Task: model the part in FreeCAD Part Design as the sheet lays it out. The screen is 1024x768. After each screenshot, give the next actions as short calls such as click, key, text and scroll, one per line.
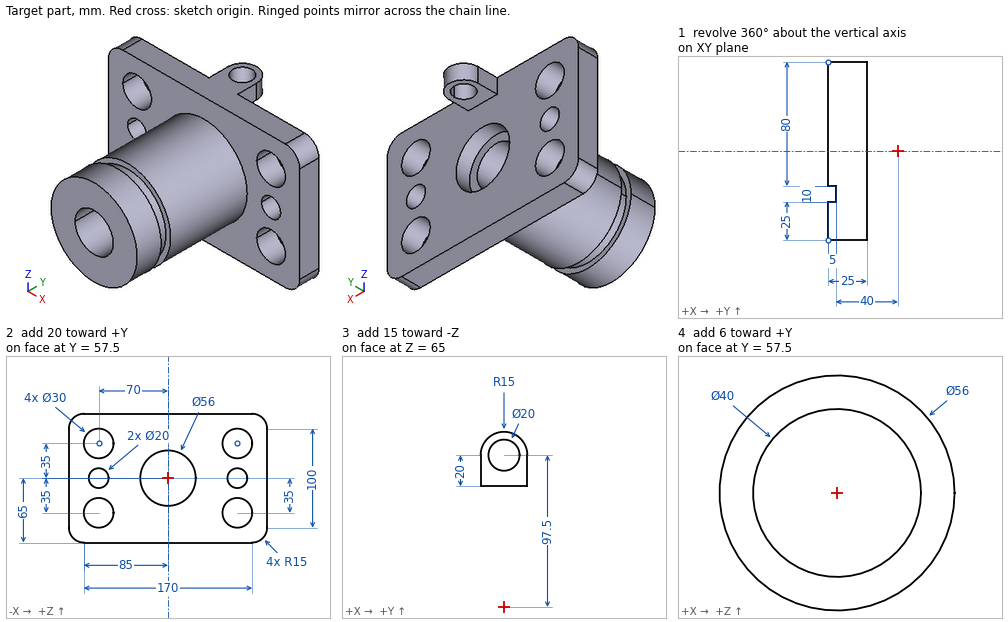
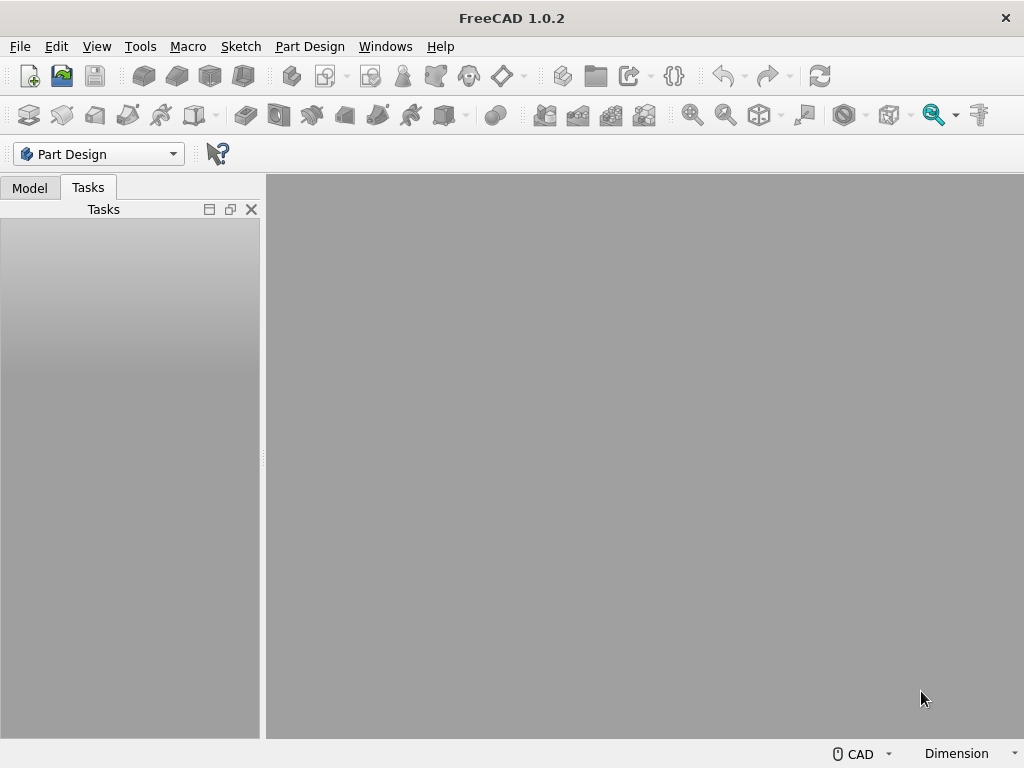
click(29, 76)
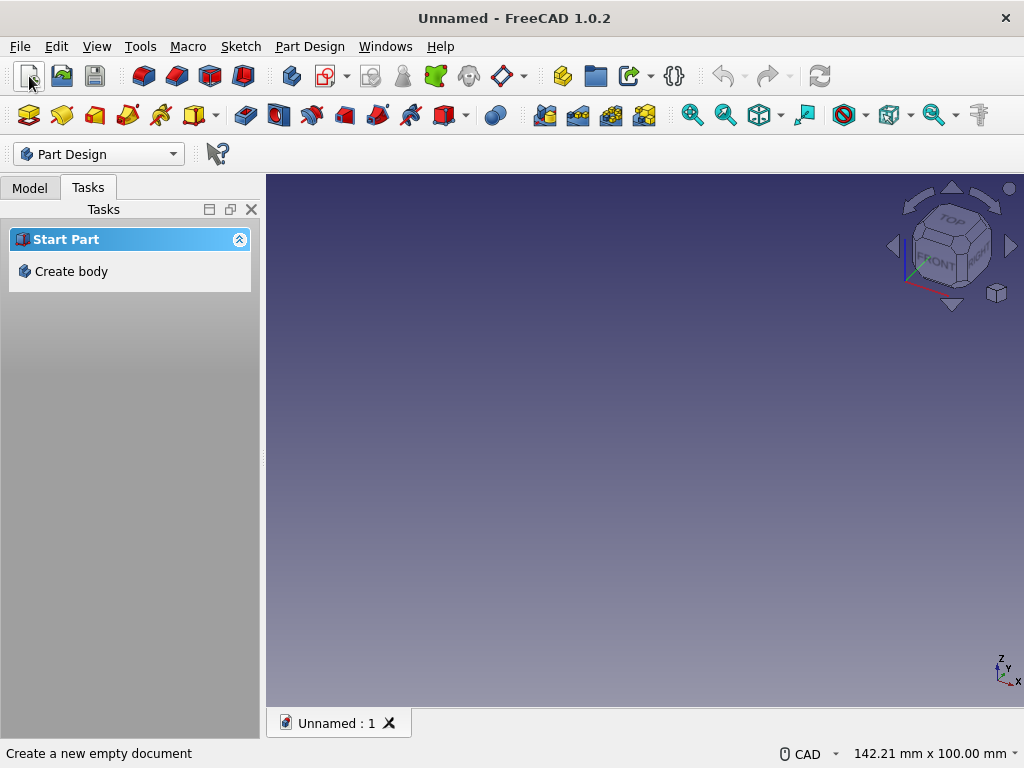
click(324, 76)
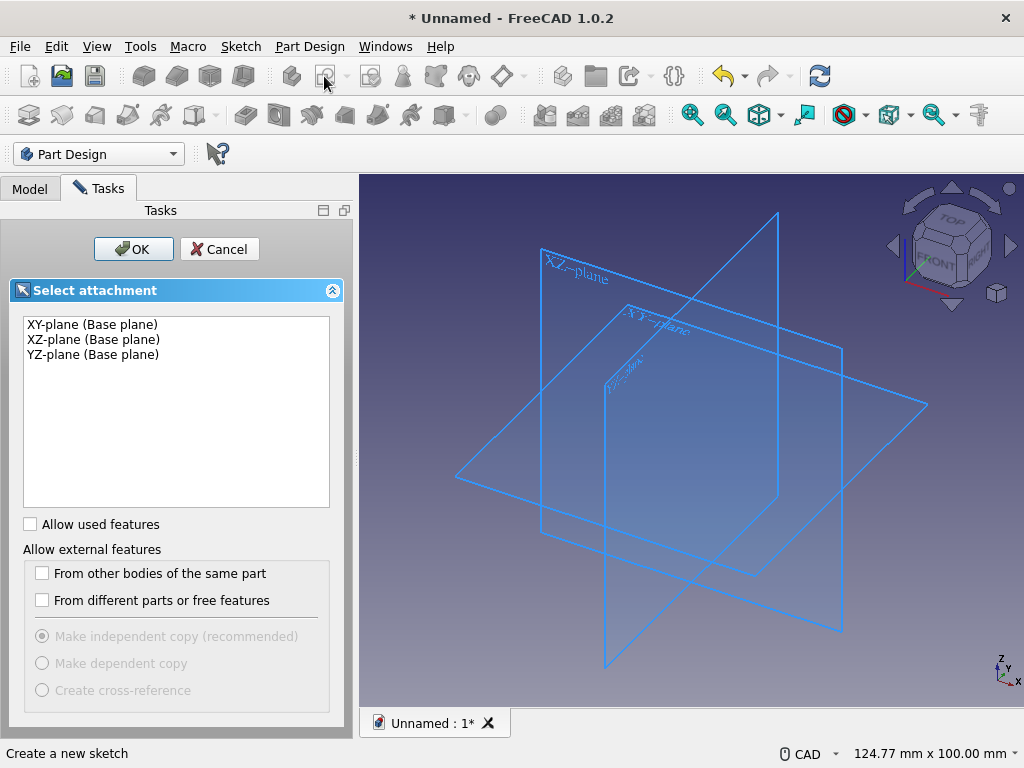
click(84, 324)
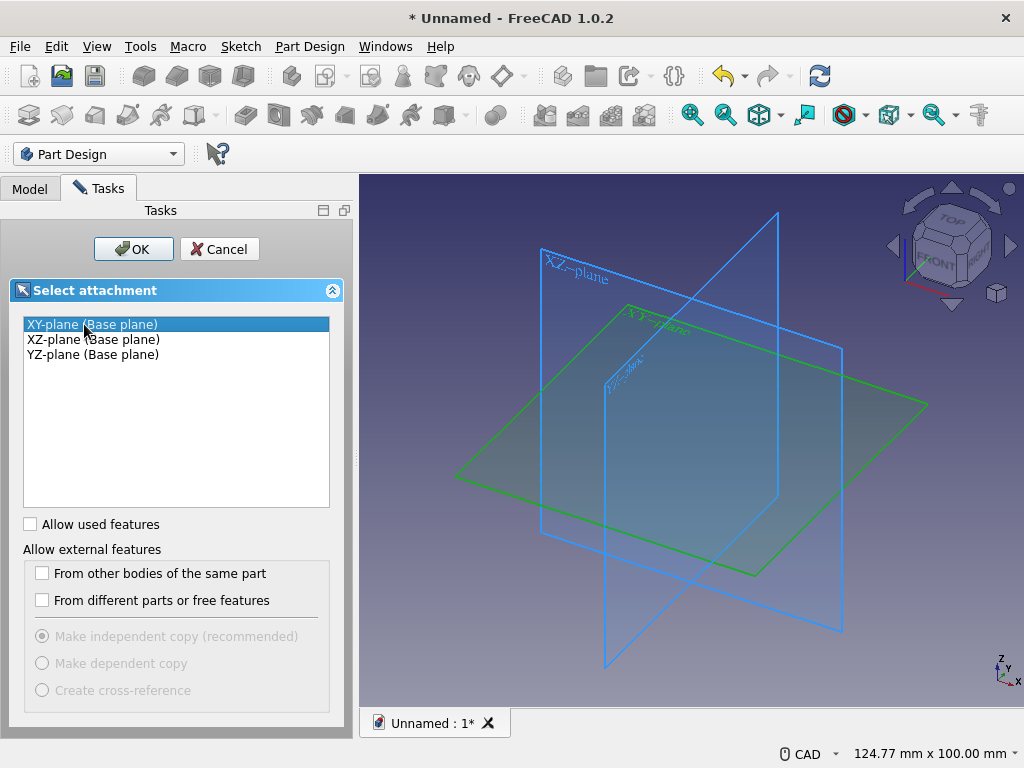
click(134, 249)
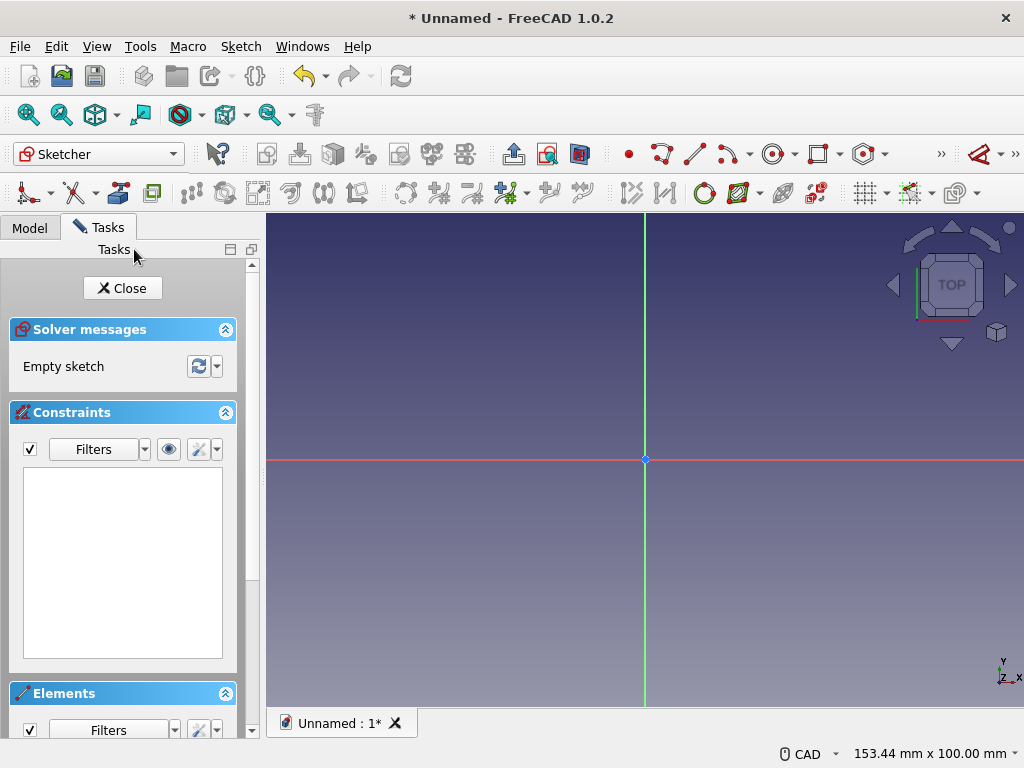
scroll(628, 460, down, 3)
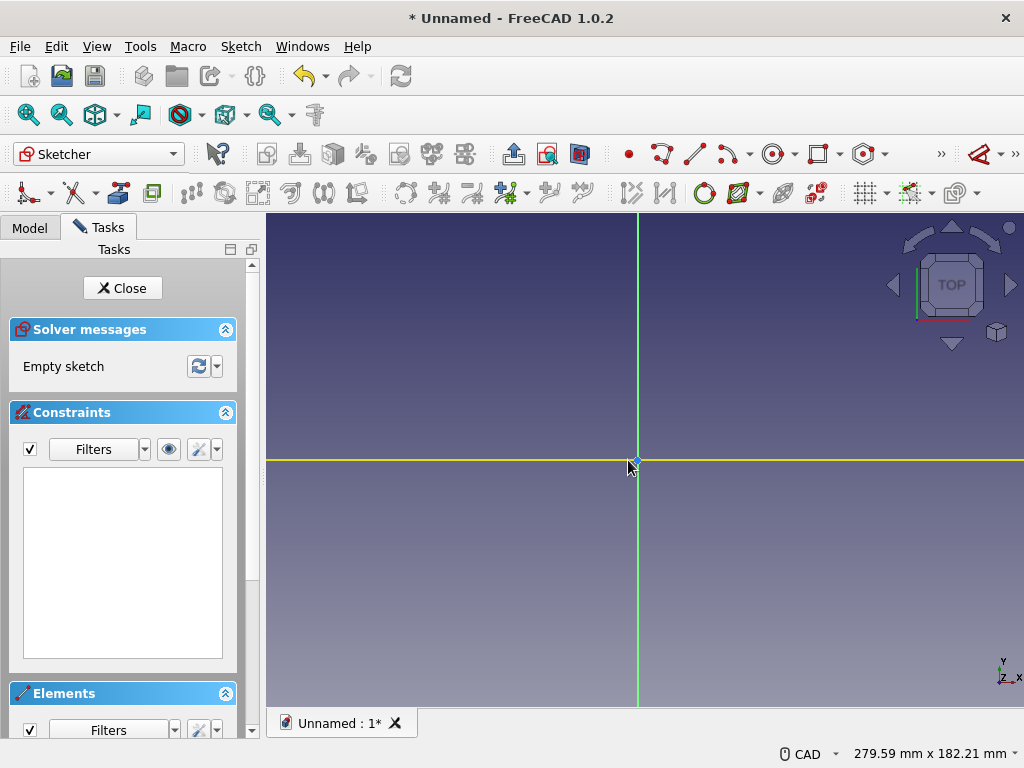
click(662, 154)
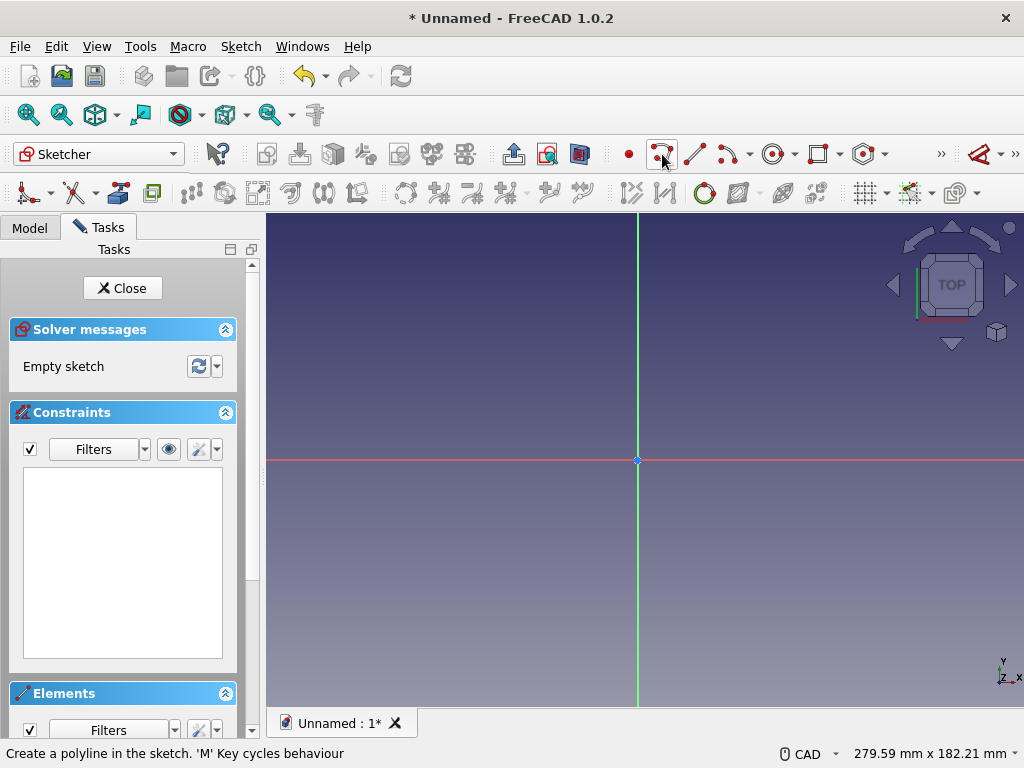
click(529, 521)
click(529, 548)
click(516, 548)
click(516, 616)
click(583, 616)
click(583, 304)
click(516, 304)
click(516, 521)
click(529, 522)
key(Escape)
key(Escape)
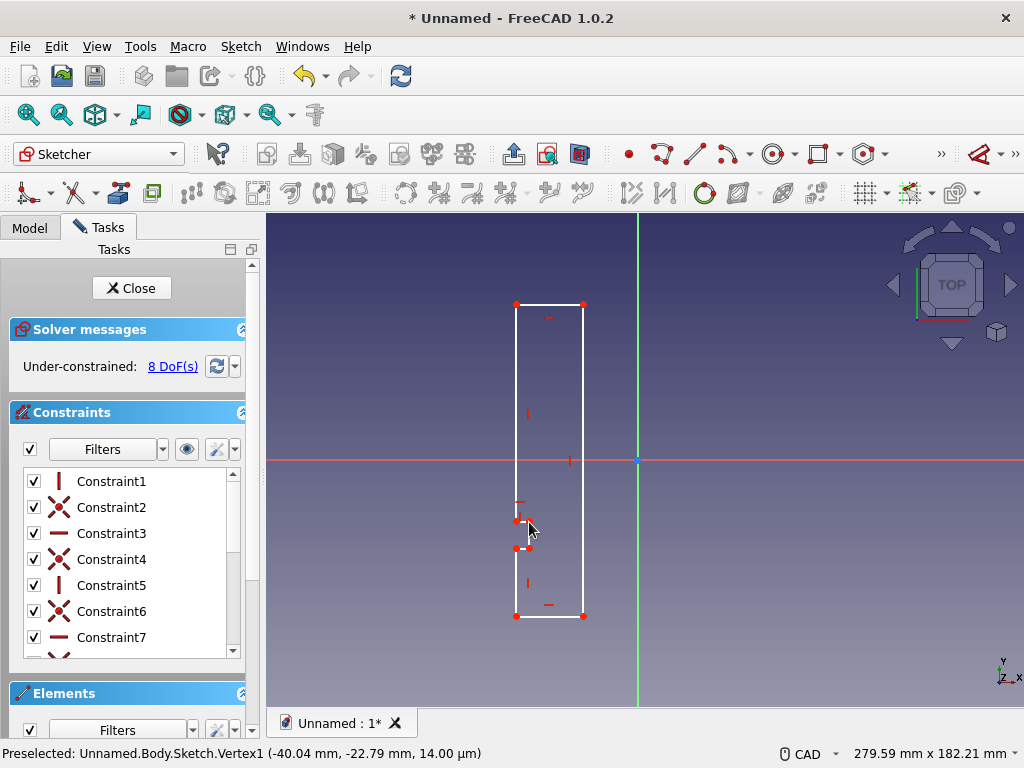
click(516, 617)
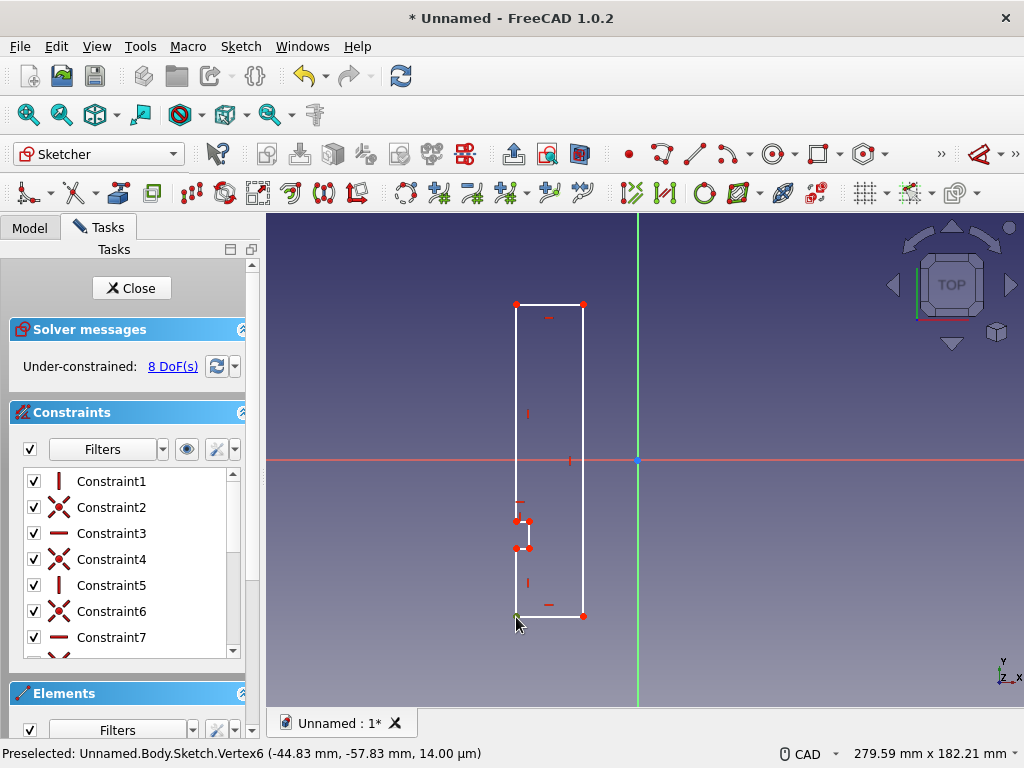
click(516, 305)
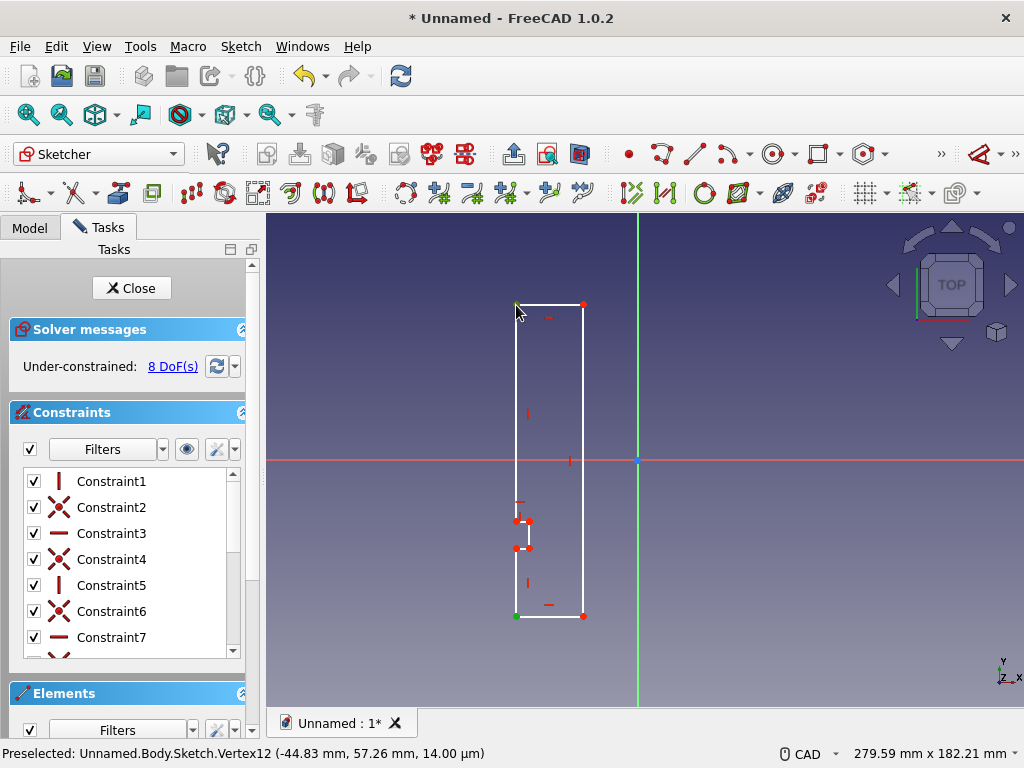
click(334, 460)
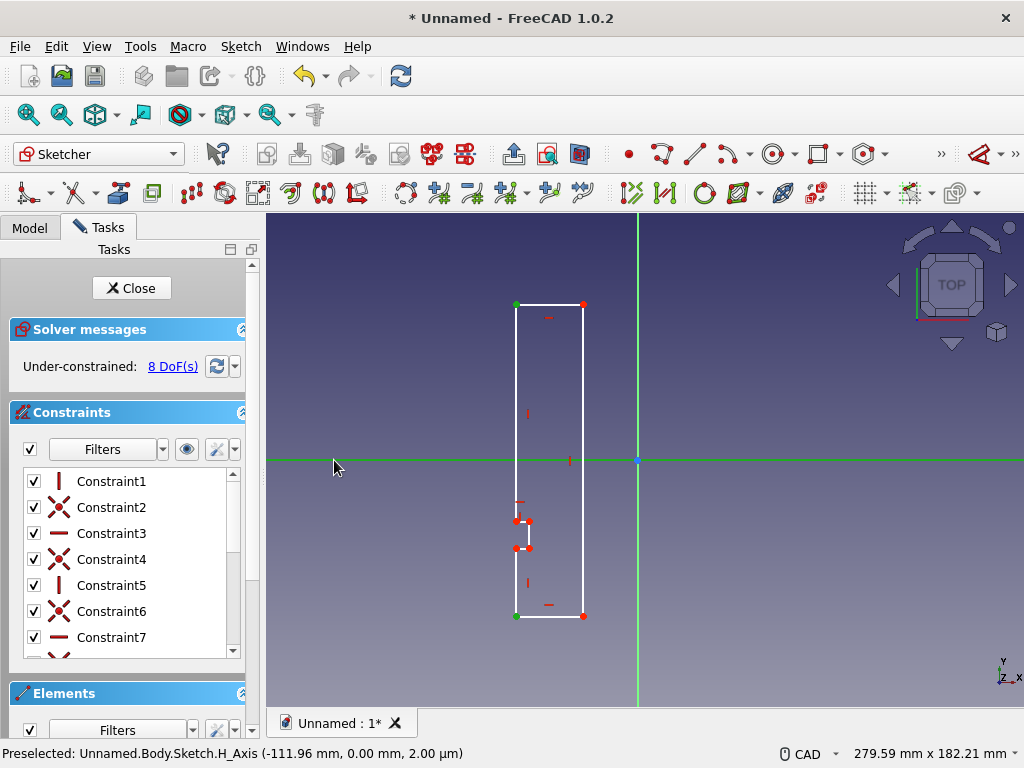
key(s)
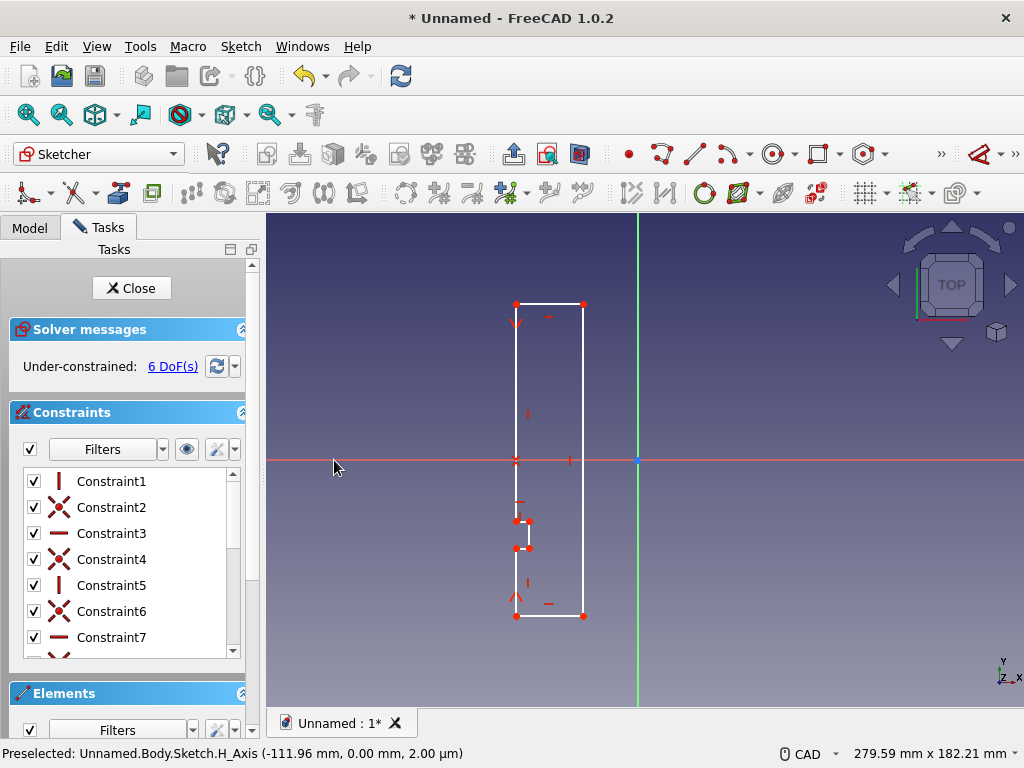
click(978, 154)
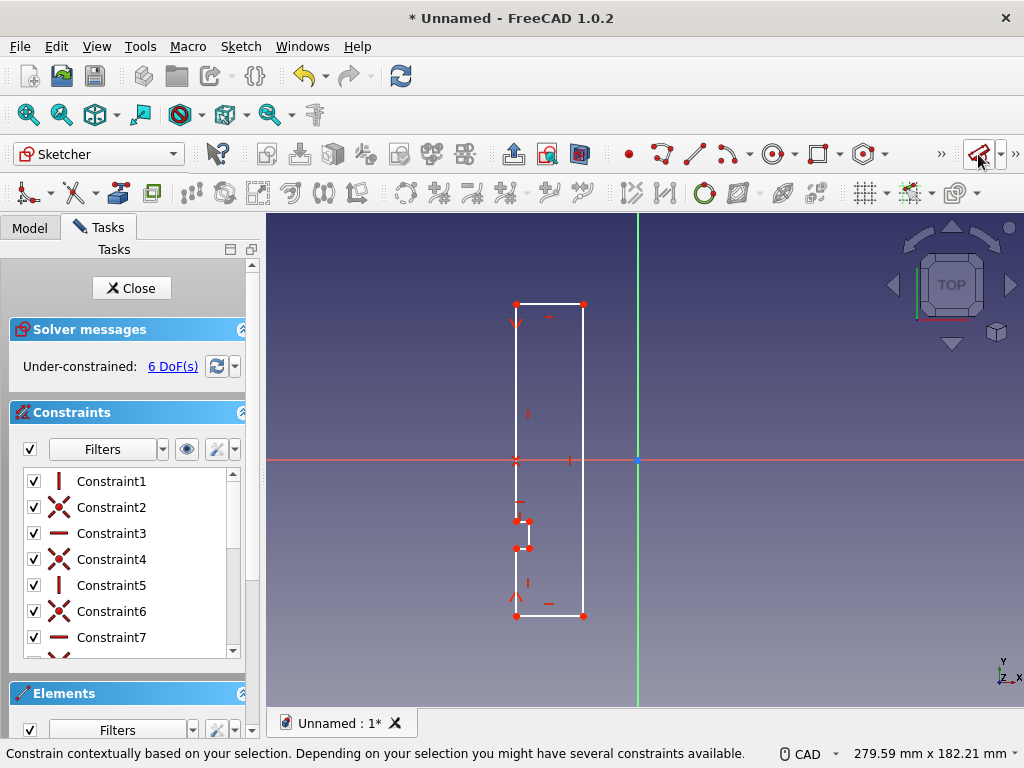
scroll(523, 549, up, 6)